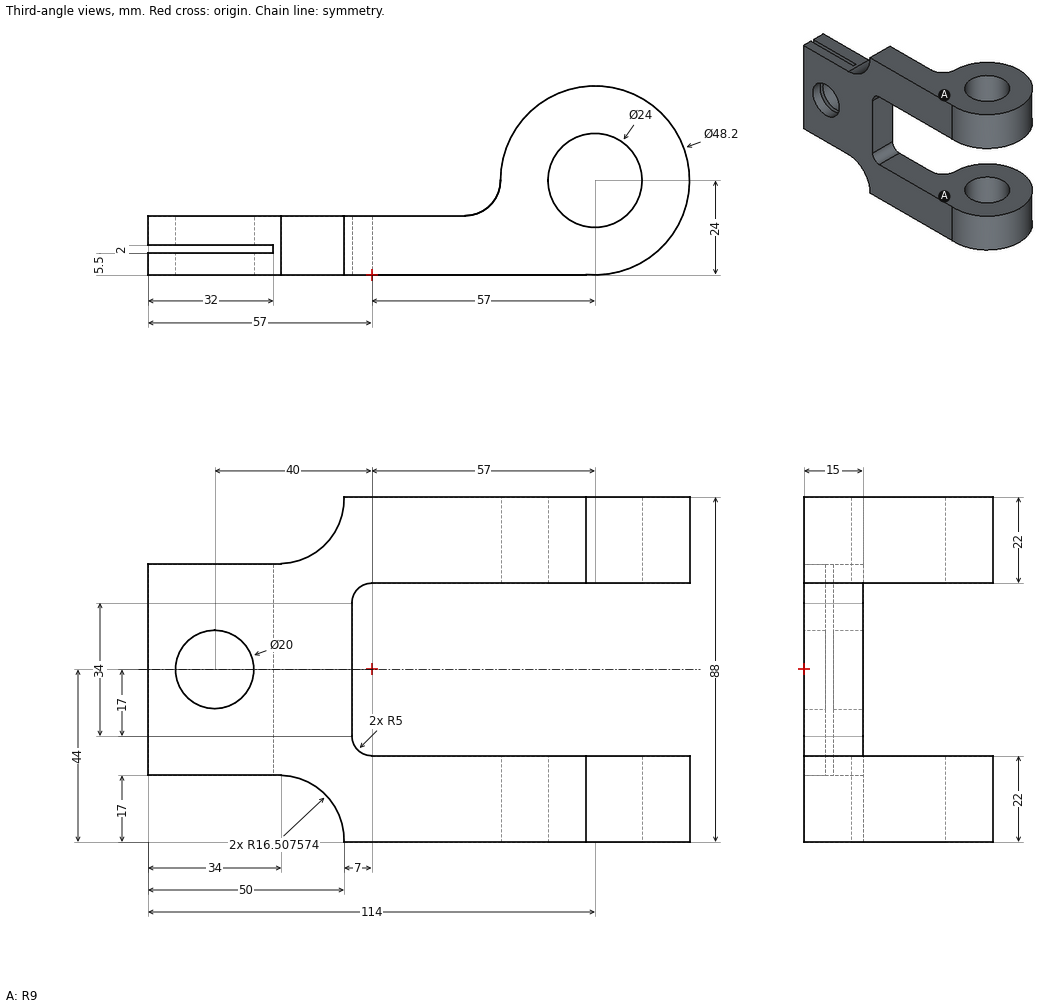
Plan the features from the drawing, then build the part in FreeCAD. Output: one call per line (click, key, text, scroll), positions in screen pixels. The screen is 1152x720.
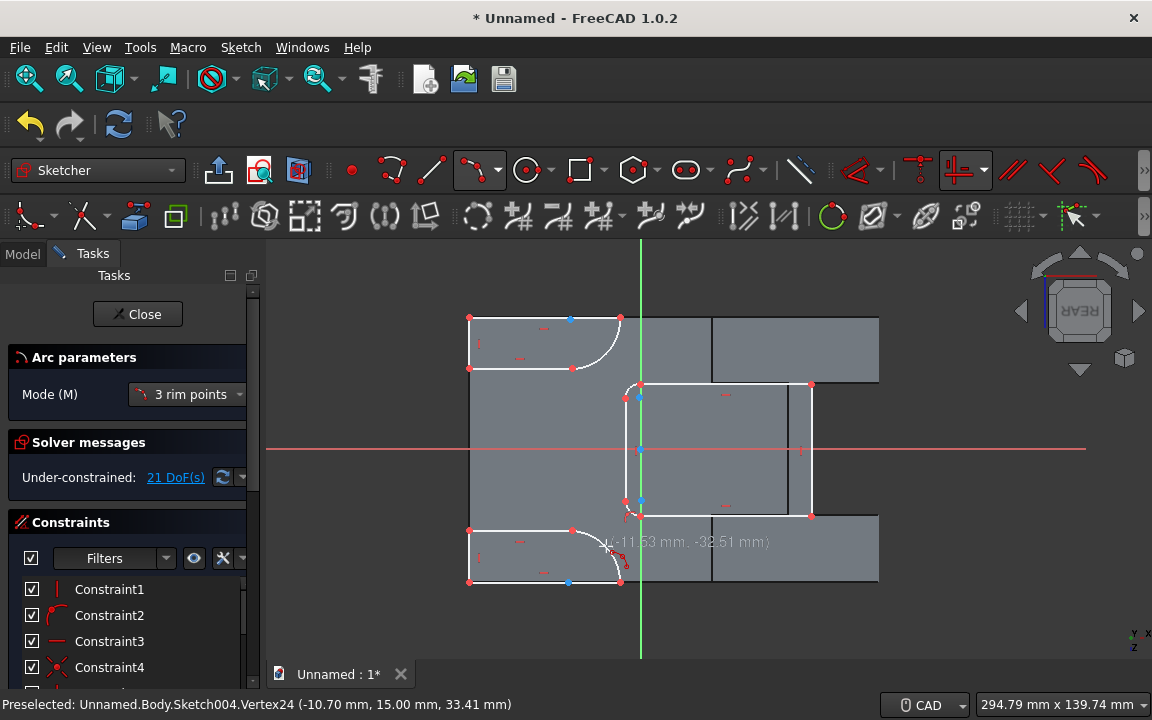
key(g)
key(c)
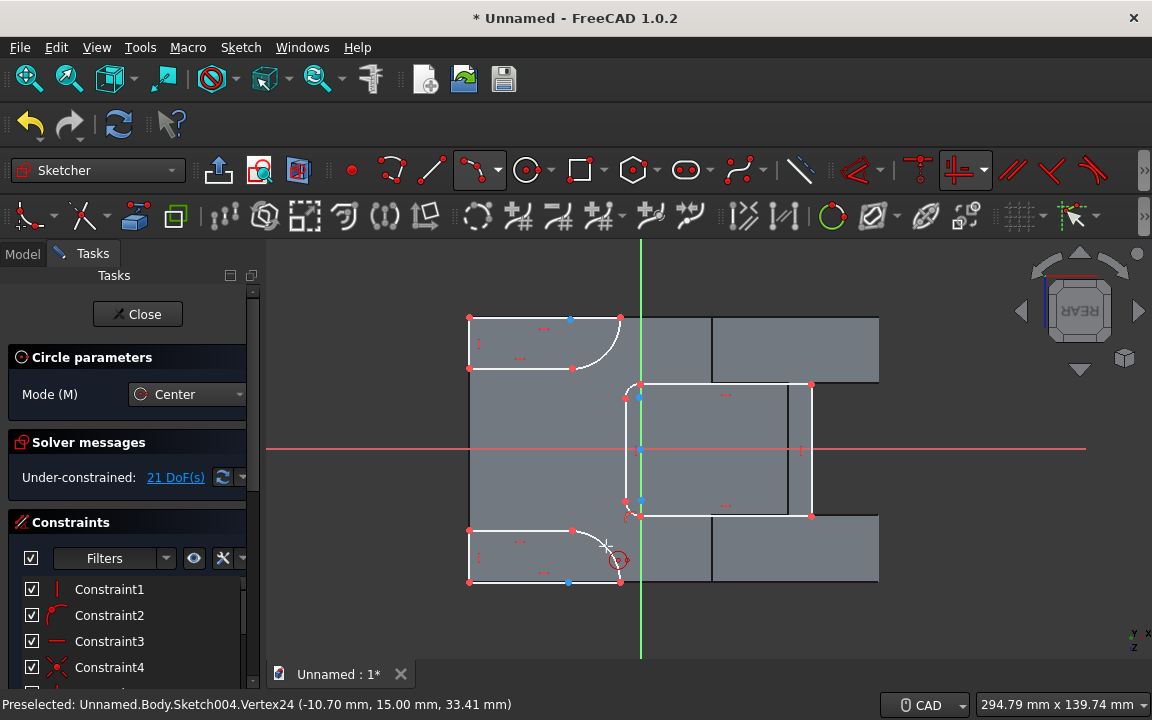
click(520, 449)
move(542, 428)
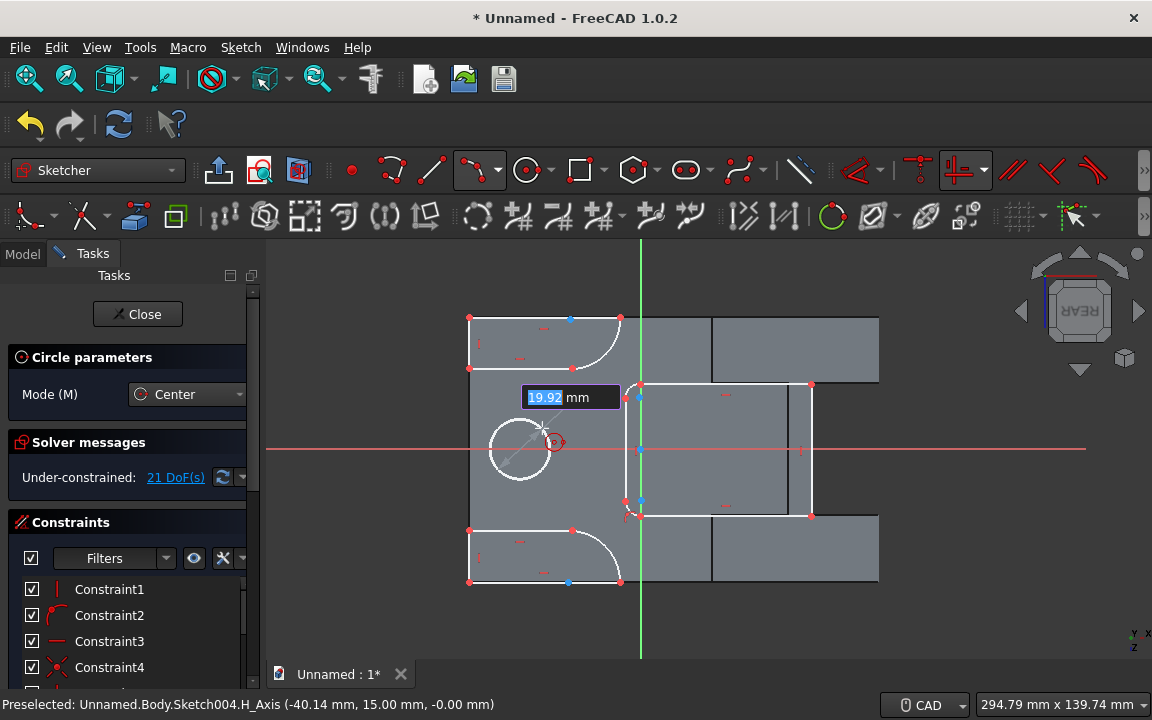
text(20)
key(Return)
key(Escape)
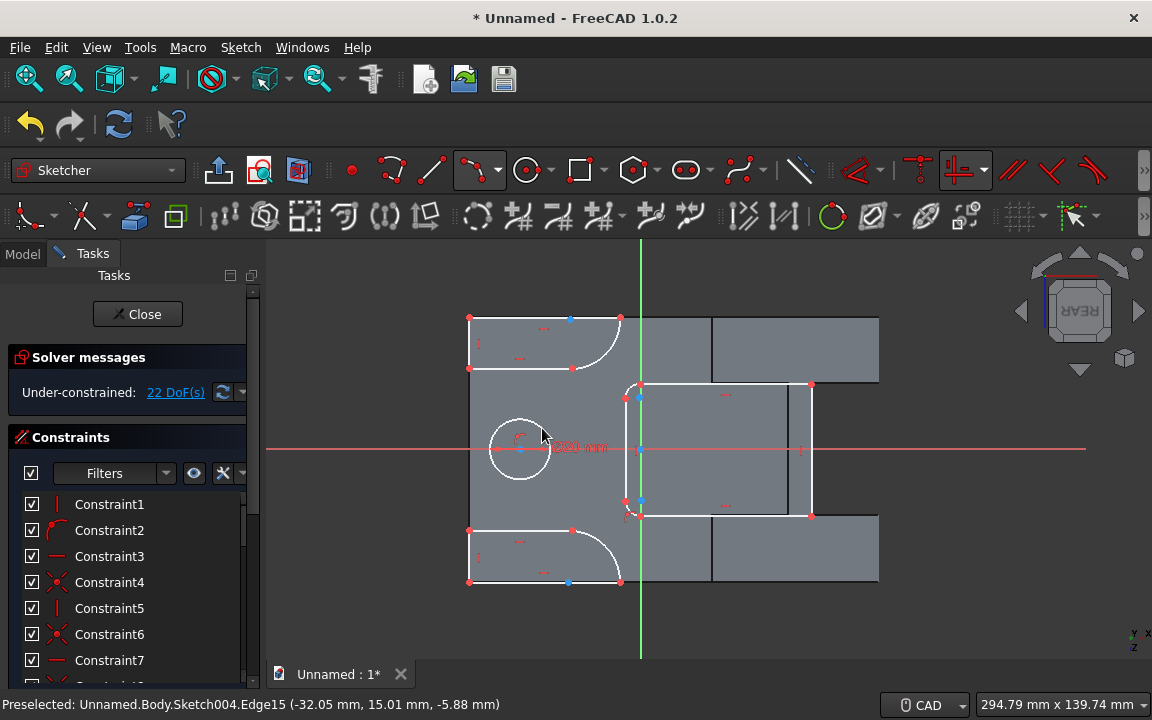
click(626, 430)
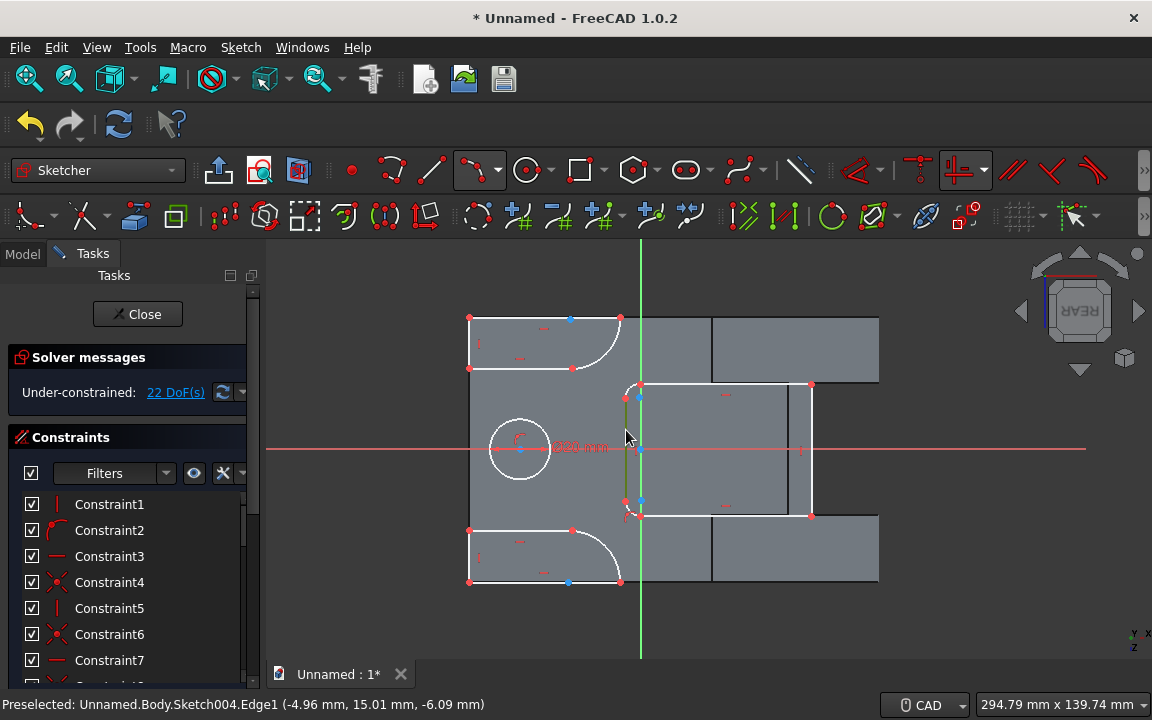
scroll(630, 512, up, 2)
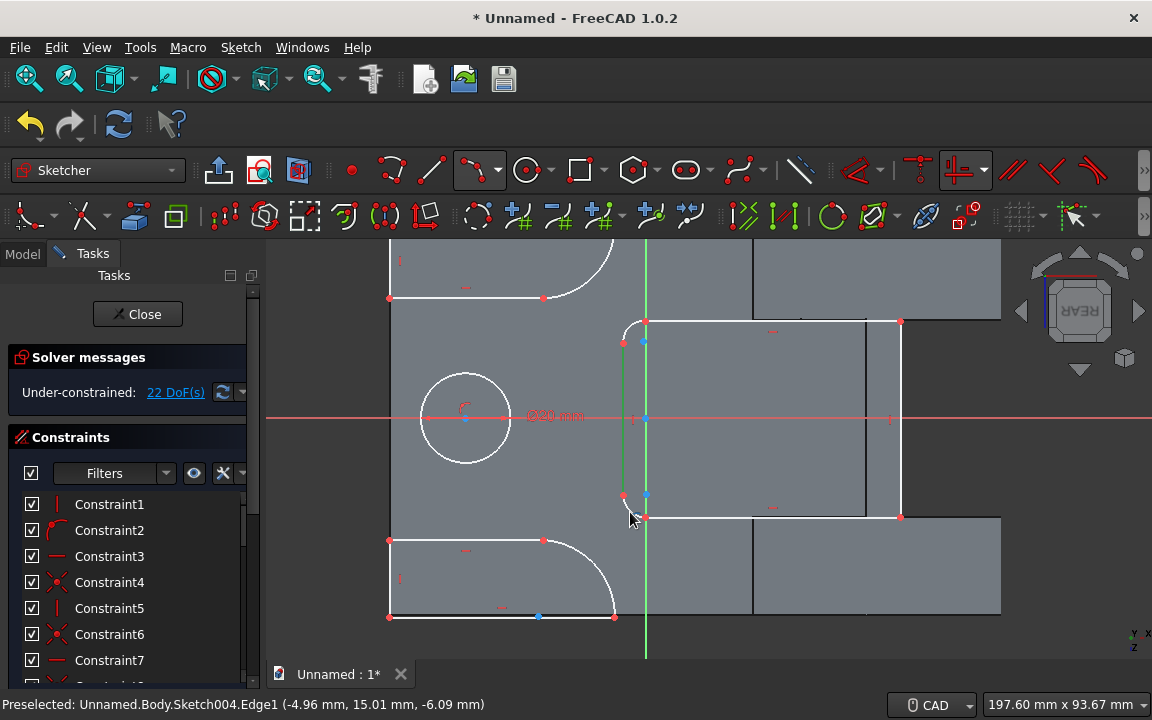
click(626, 506)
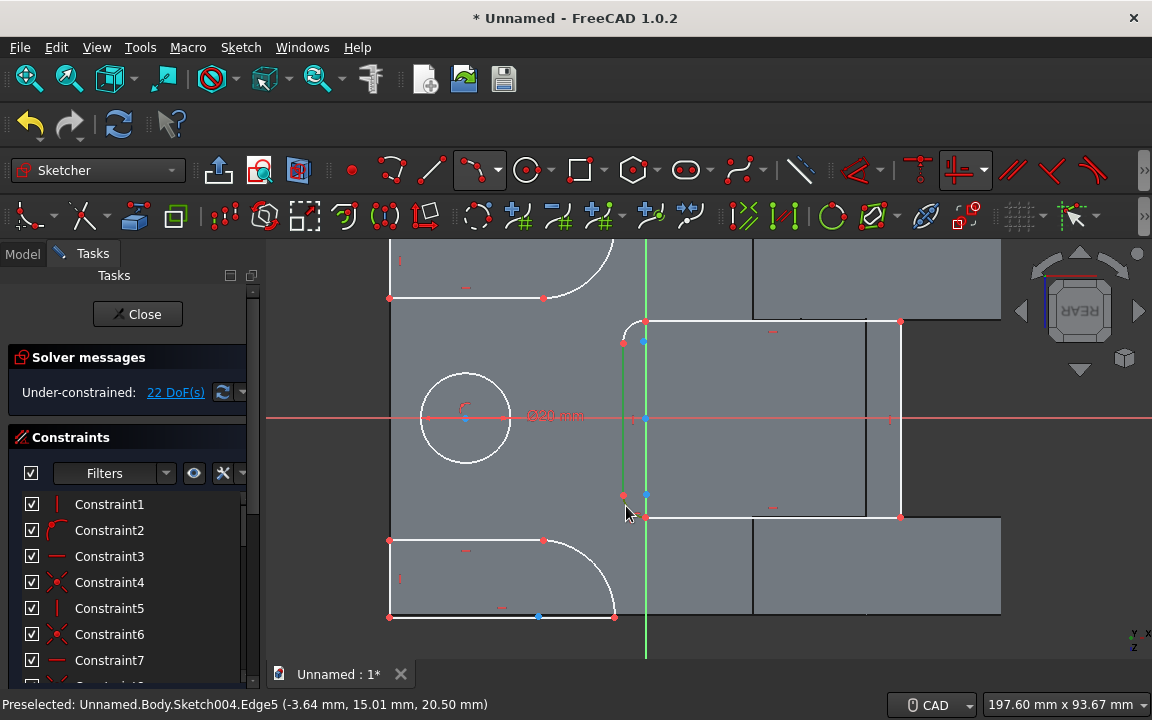
click(1094, 170)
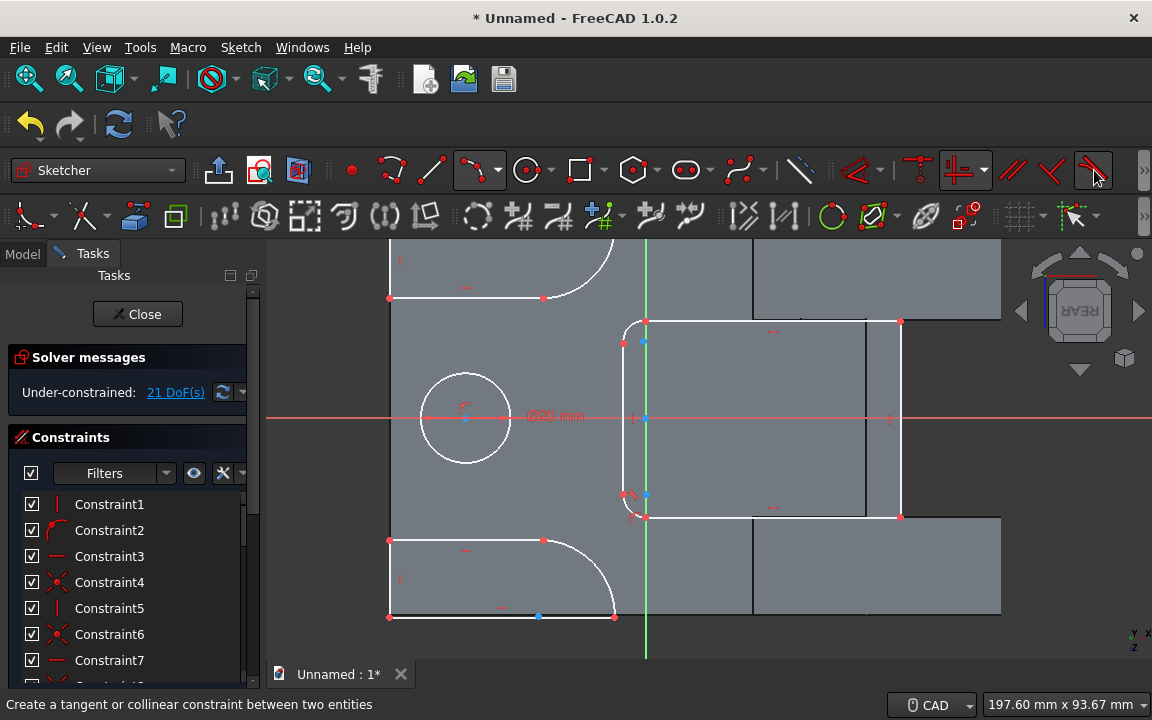
click(623, 389)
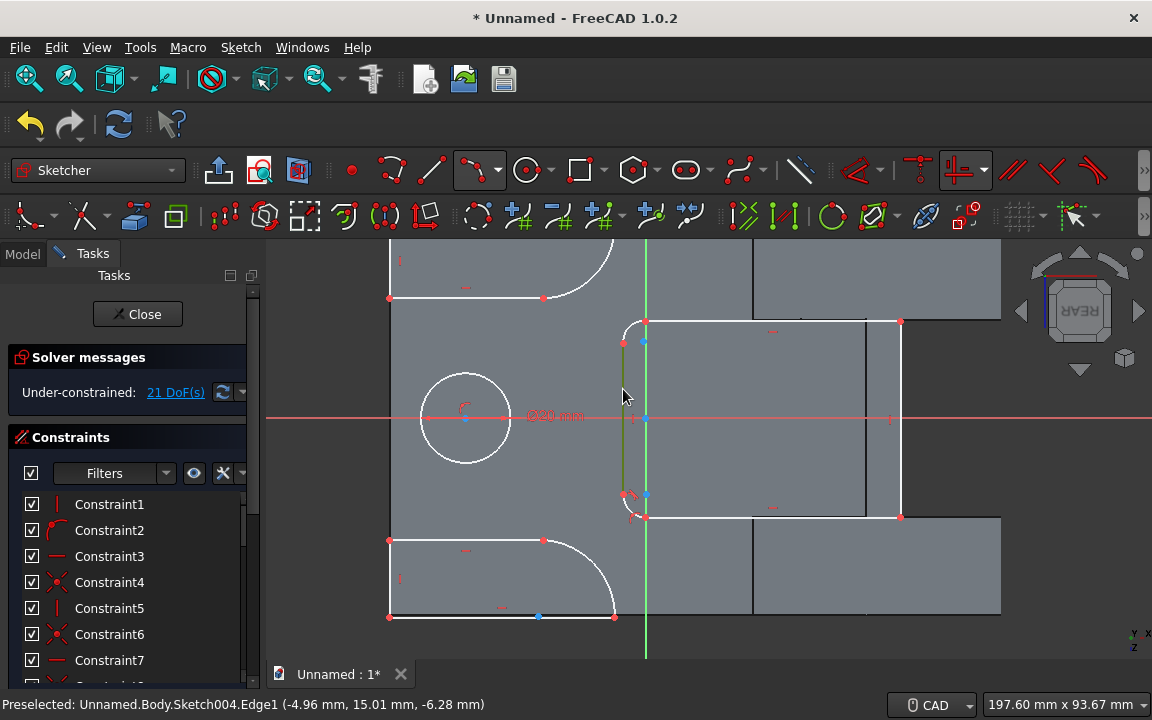
scroll(635, 323, up, 2)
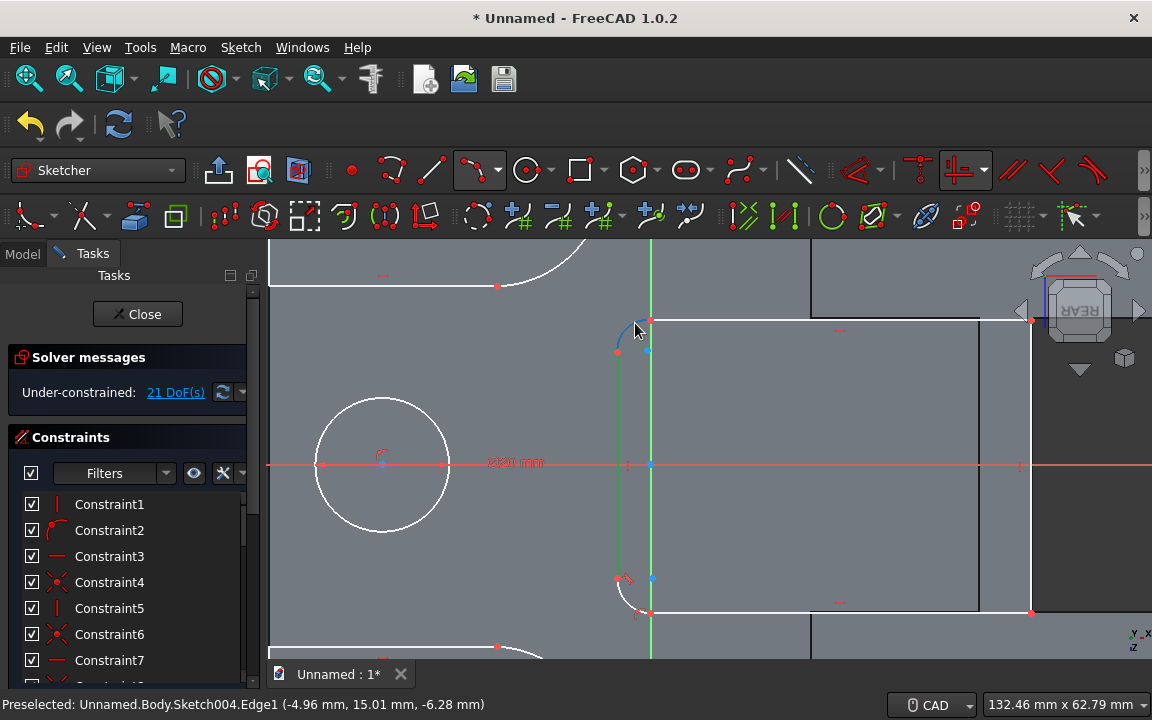
click(635, 323)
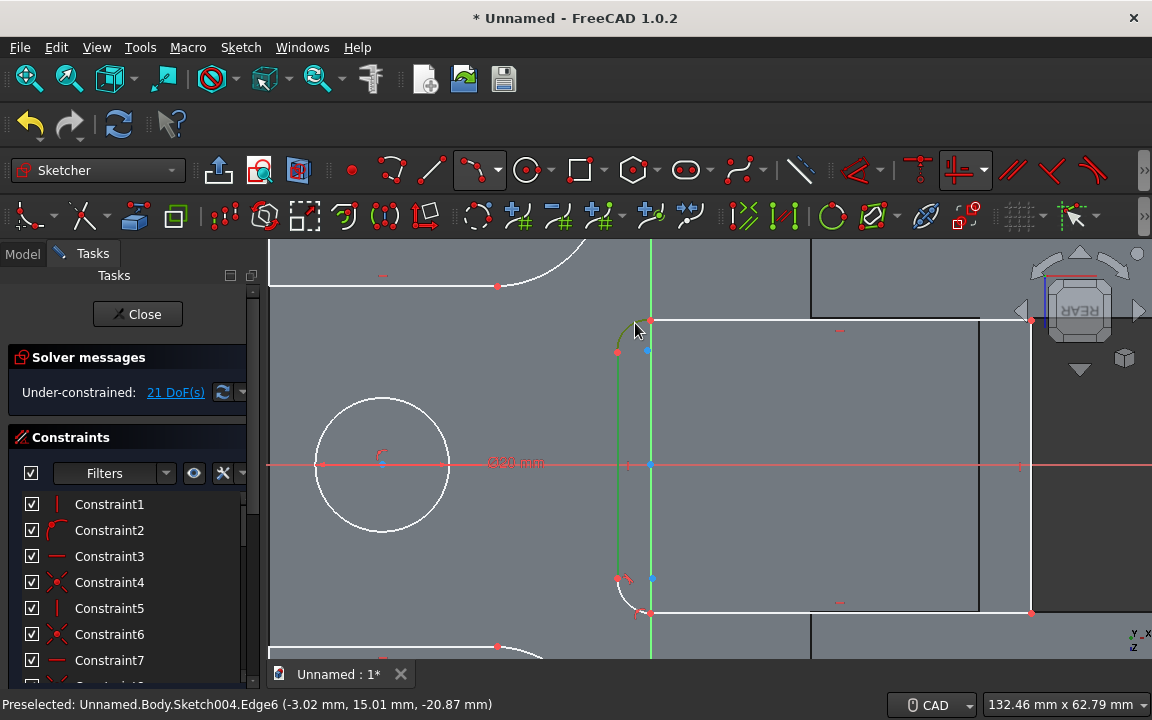
click(1094, 170)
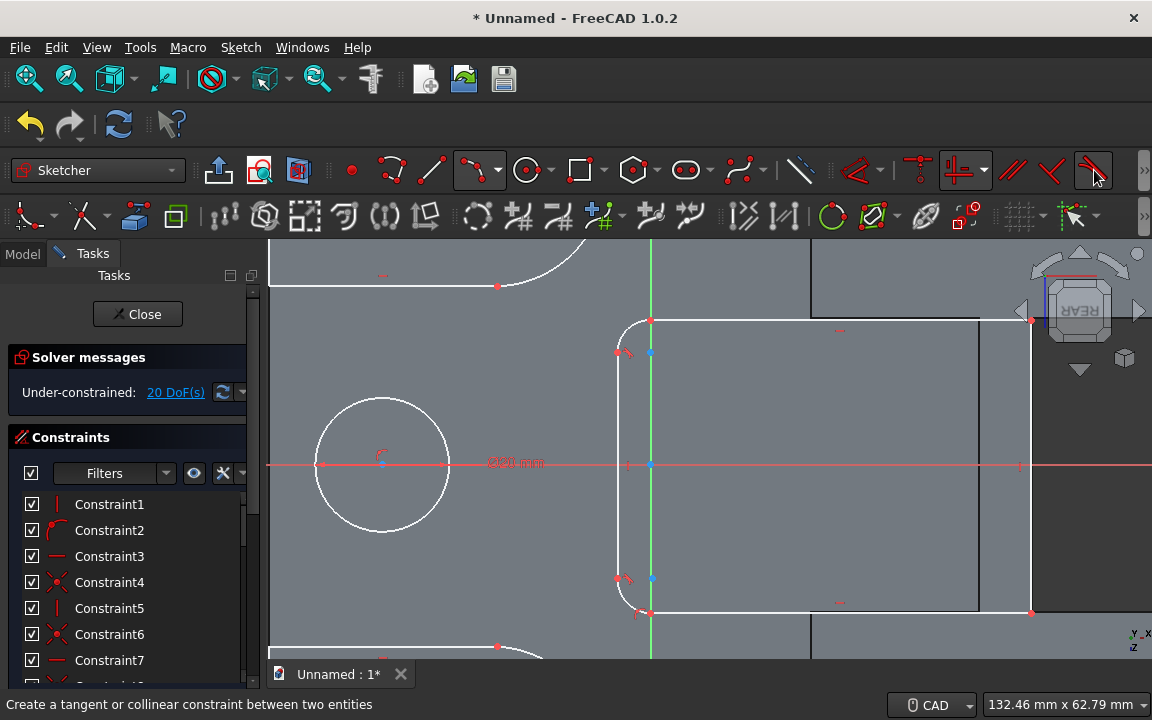
click(765, 613)